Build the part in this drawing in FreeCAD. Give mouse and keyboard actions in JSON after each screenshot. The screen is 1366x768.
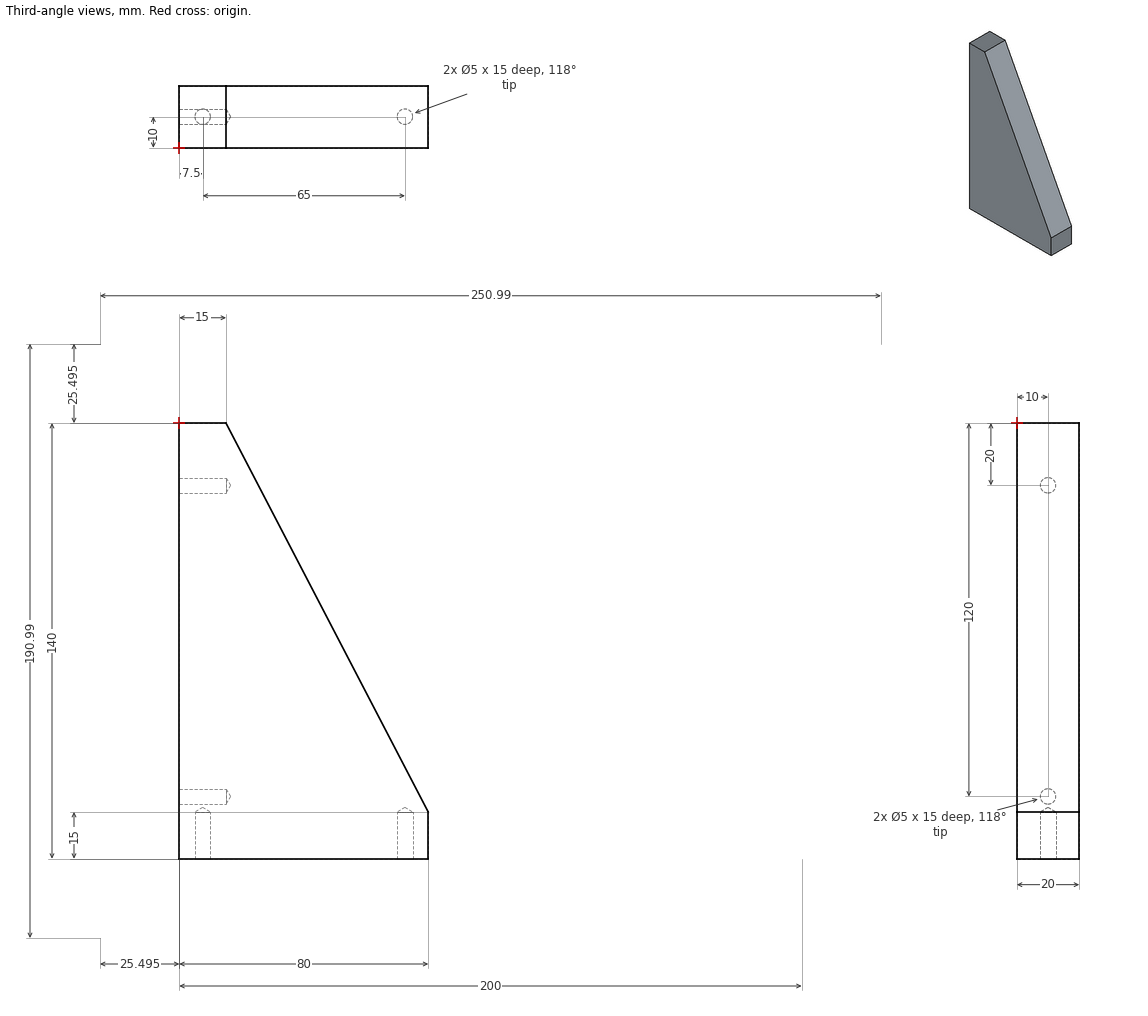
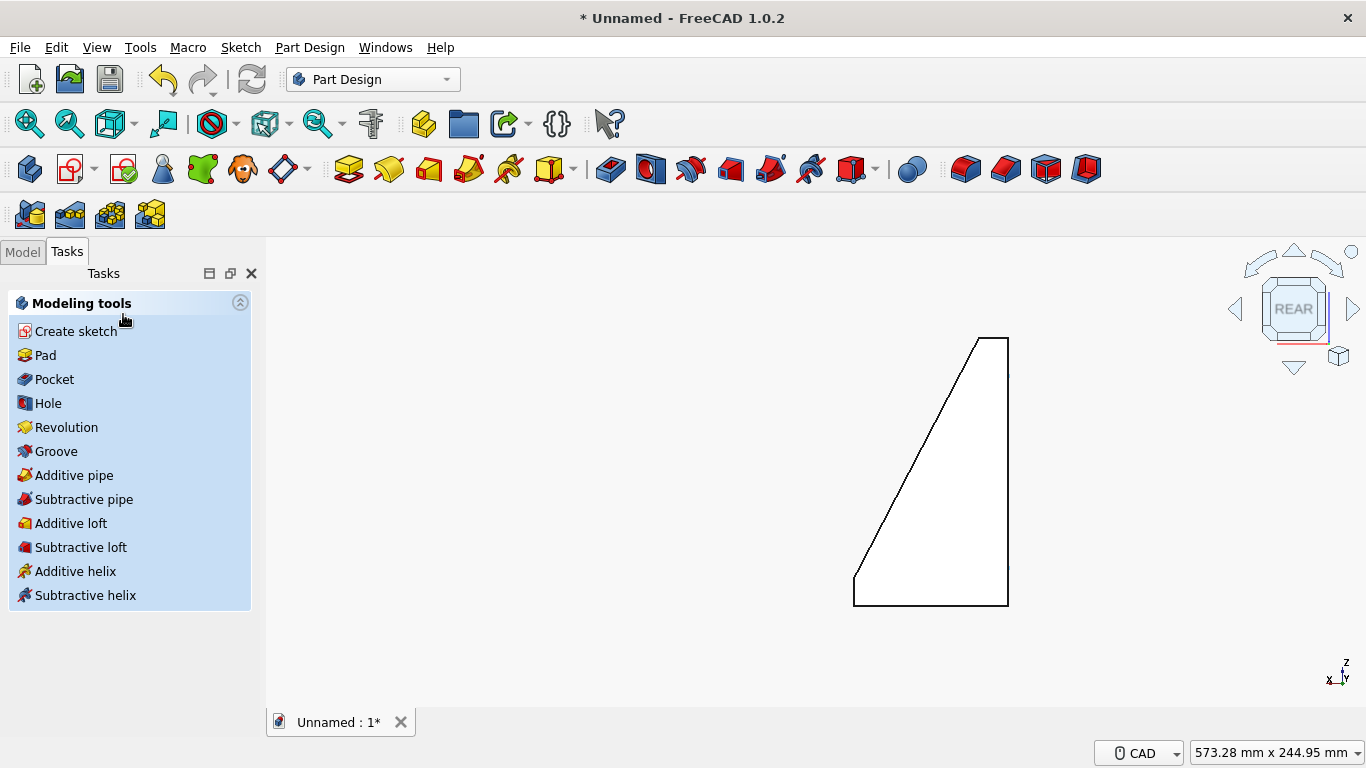
{"action": "left_click", "coordinate": [652, 170]}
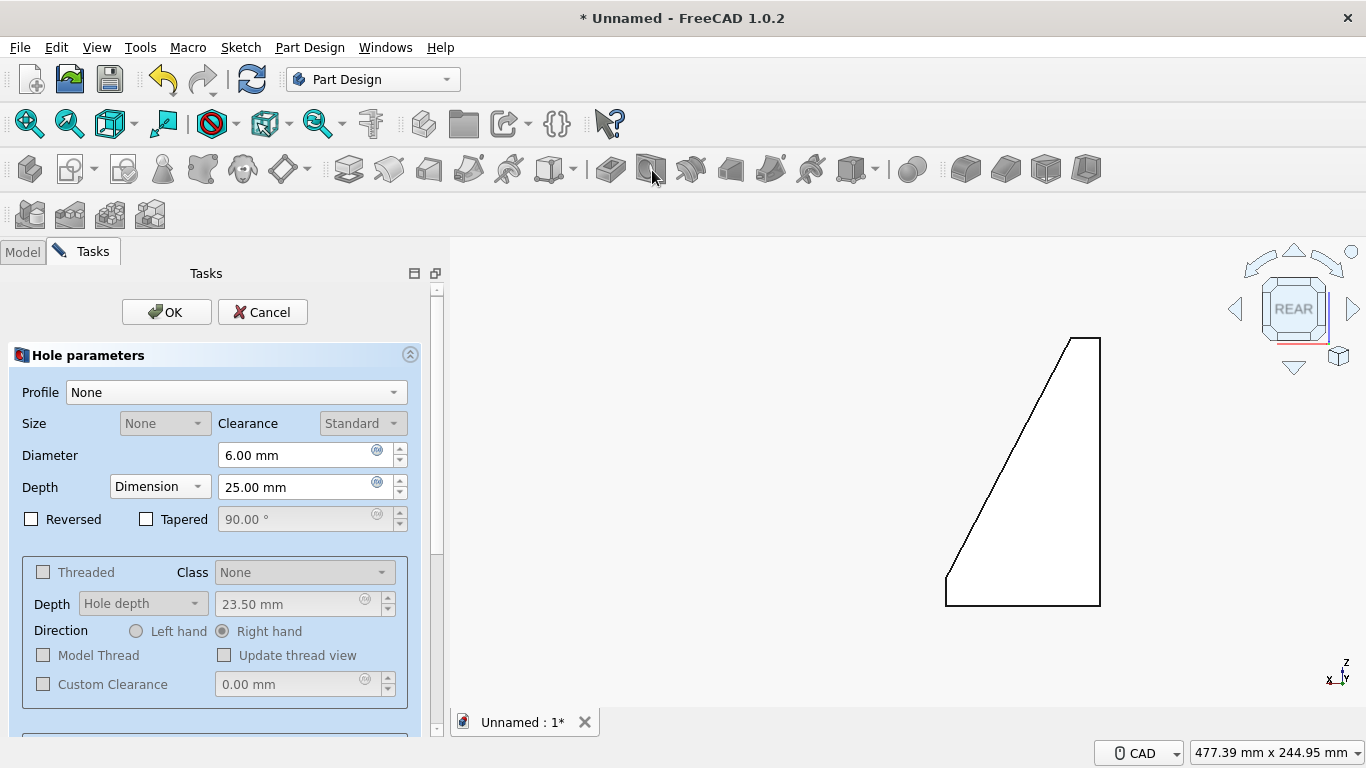
{"action": "triple_click", "coordinate": [305, 455]}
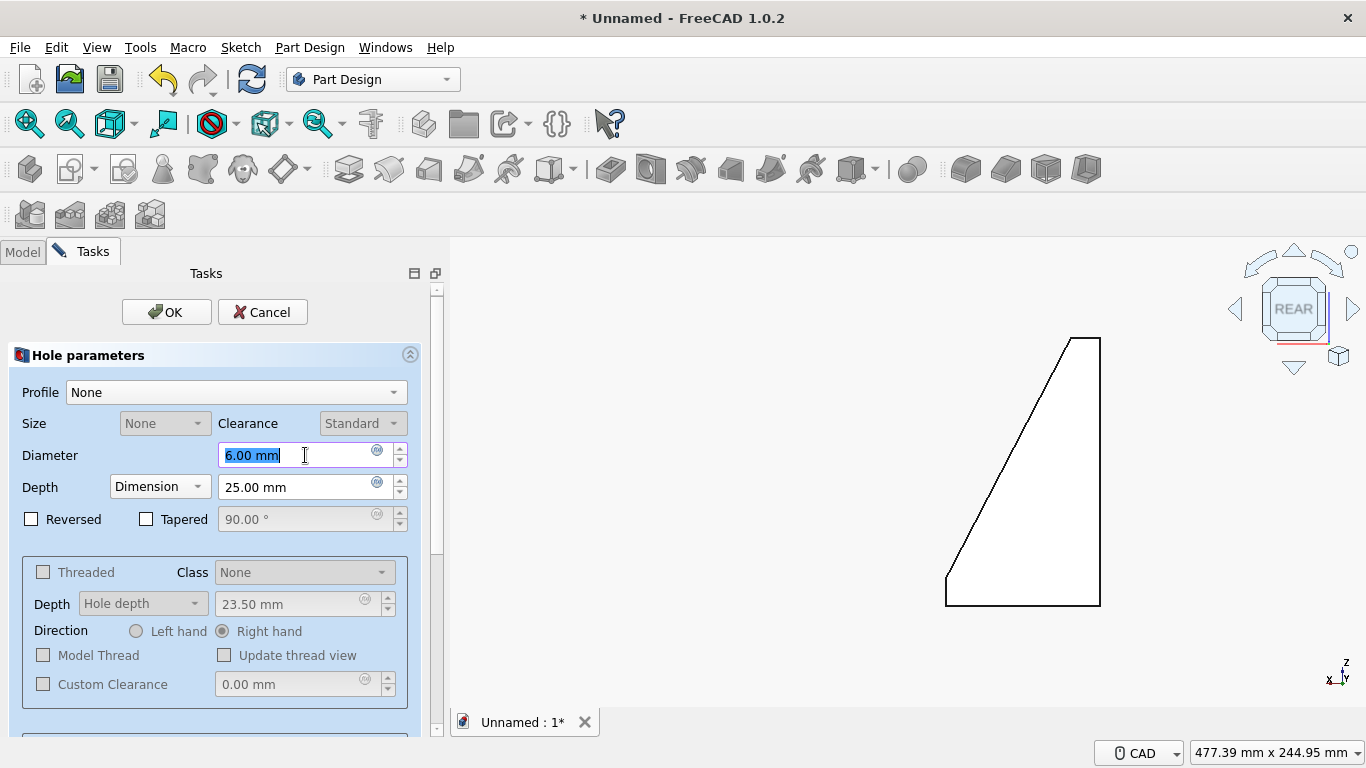
{"action": "type", "text": "5"}
{"action": "key", "text": "Tab"}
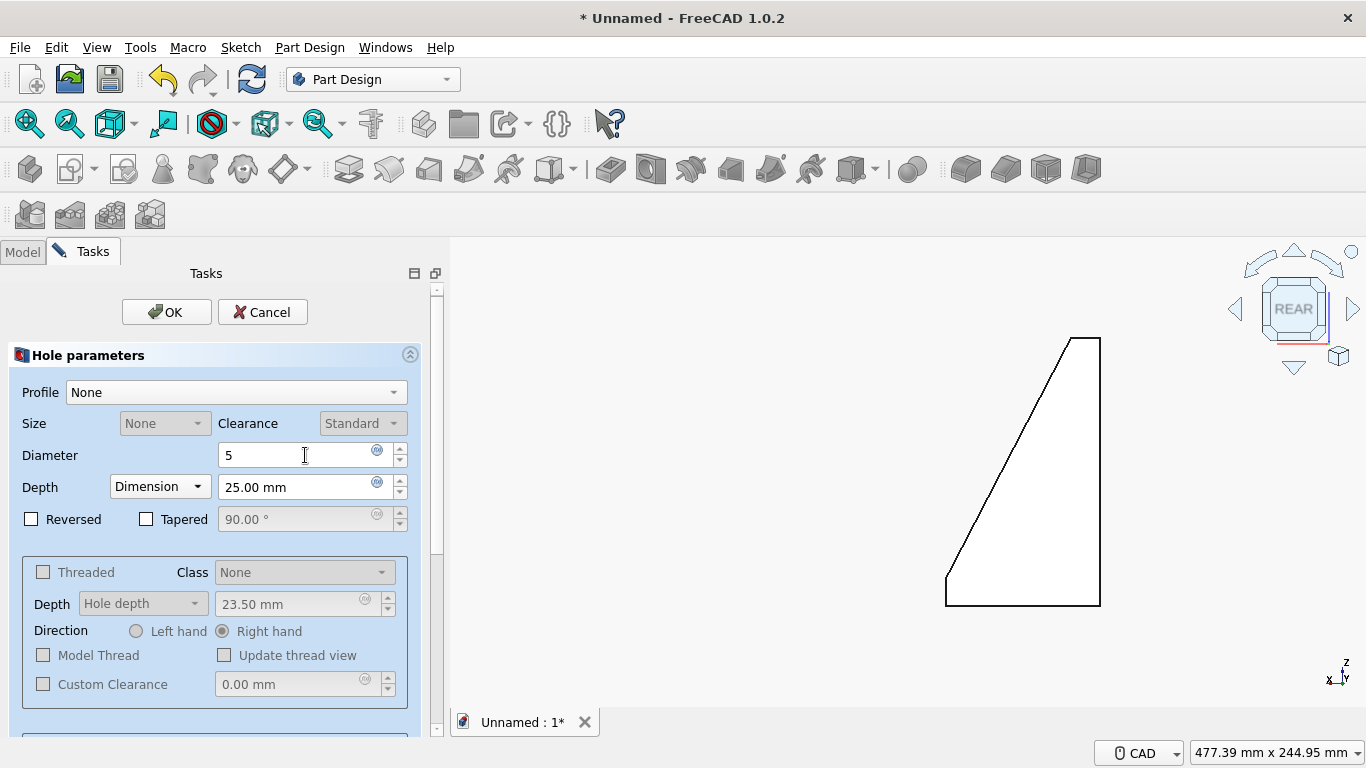
{"action": "triple_click", "coordinate": [305, 487]}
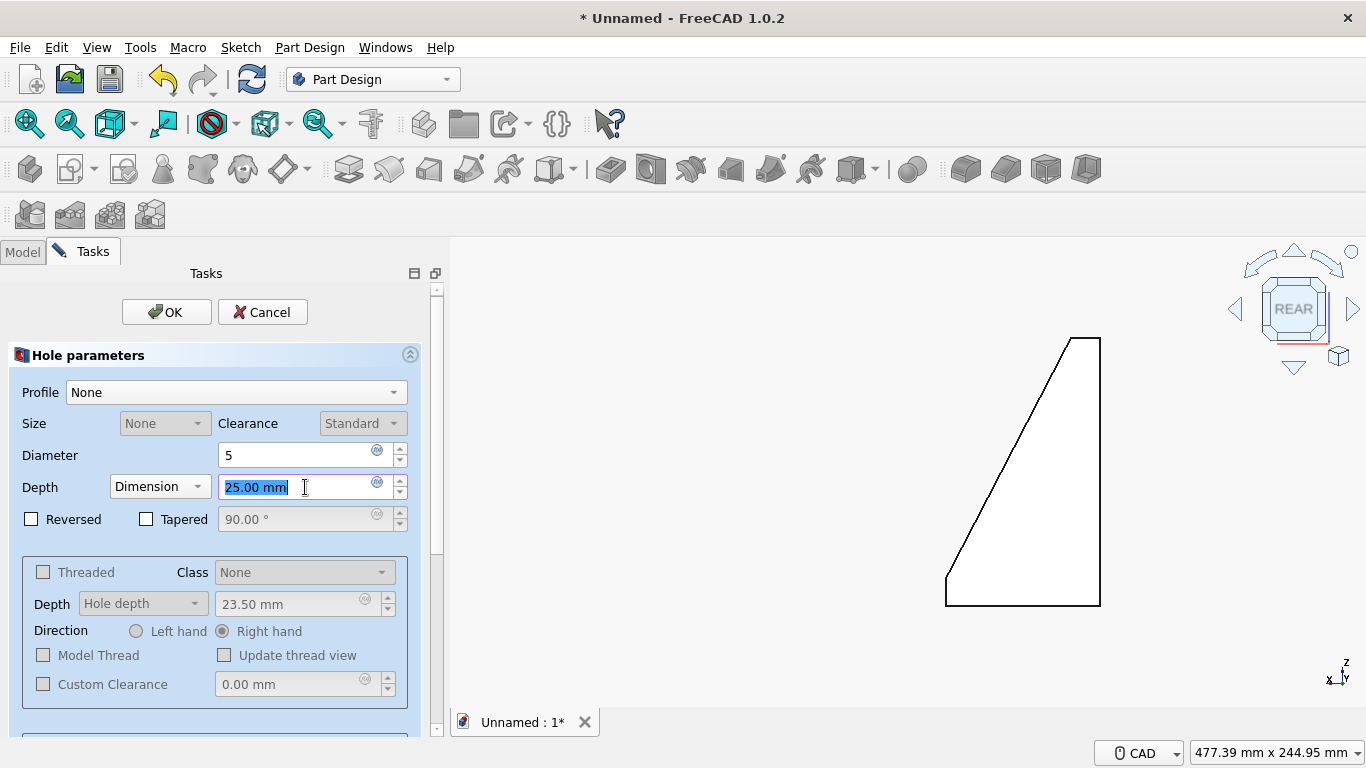
{"action": "type", "text": "15"}
{"action": "key", "text": "Tab"}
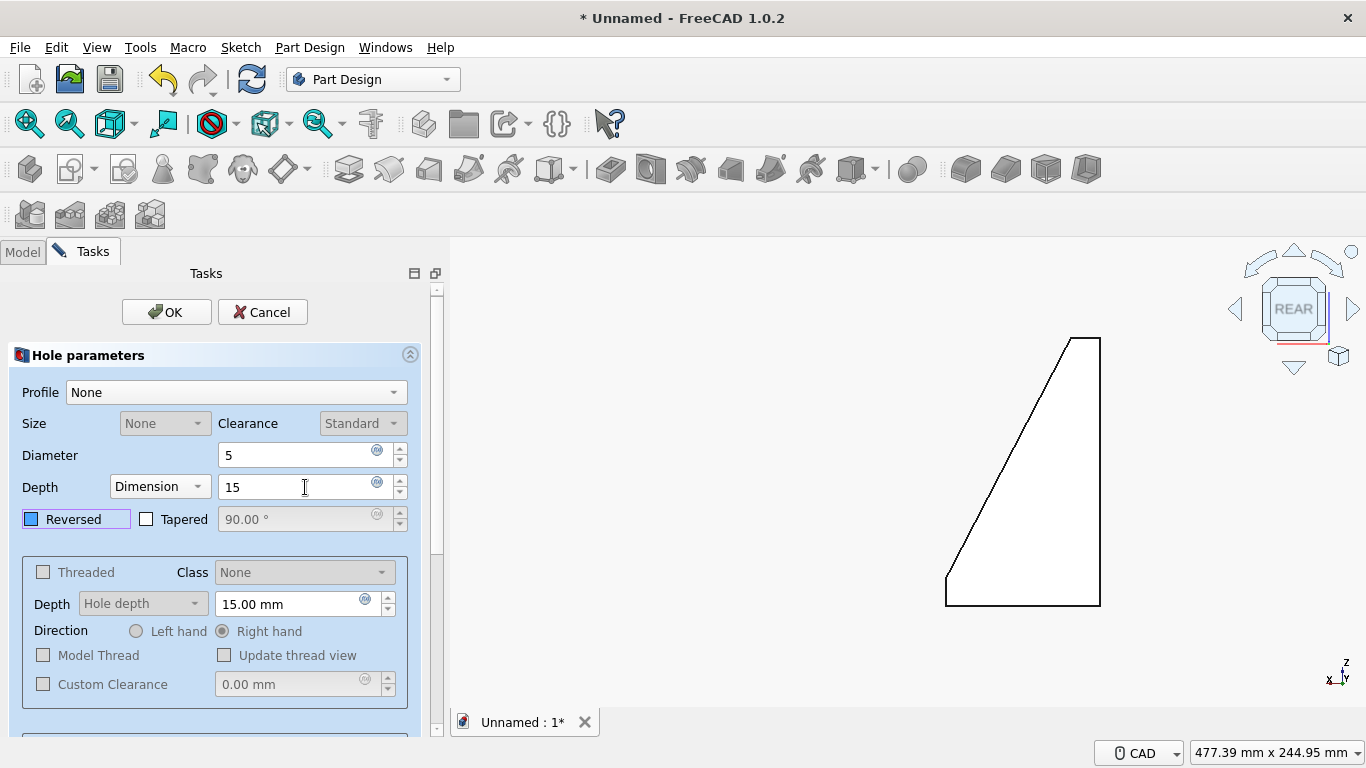
{"action": "left_click", "coordinate": [30, 519]}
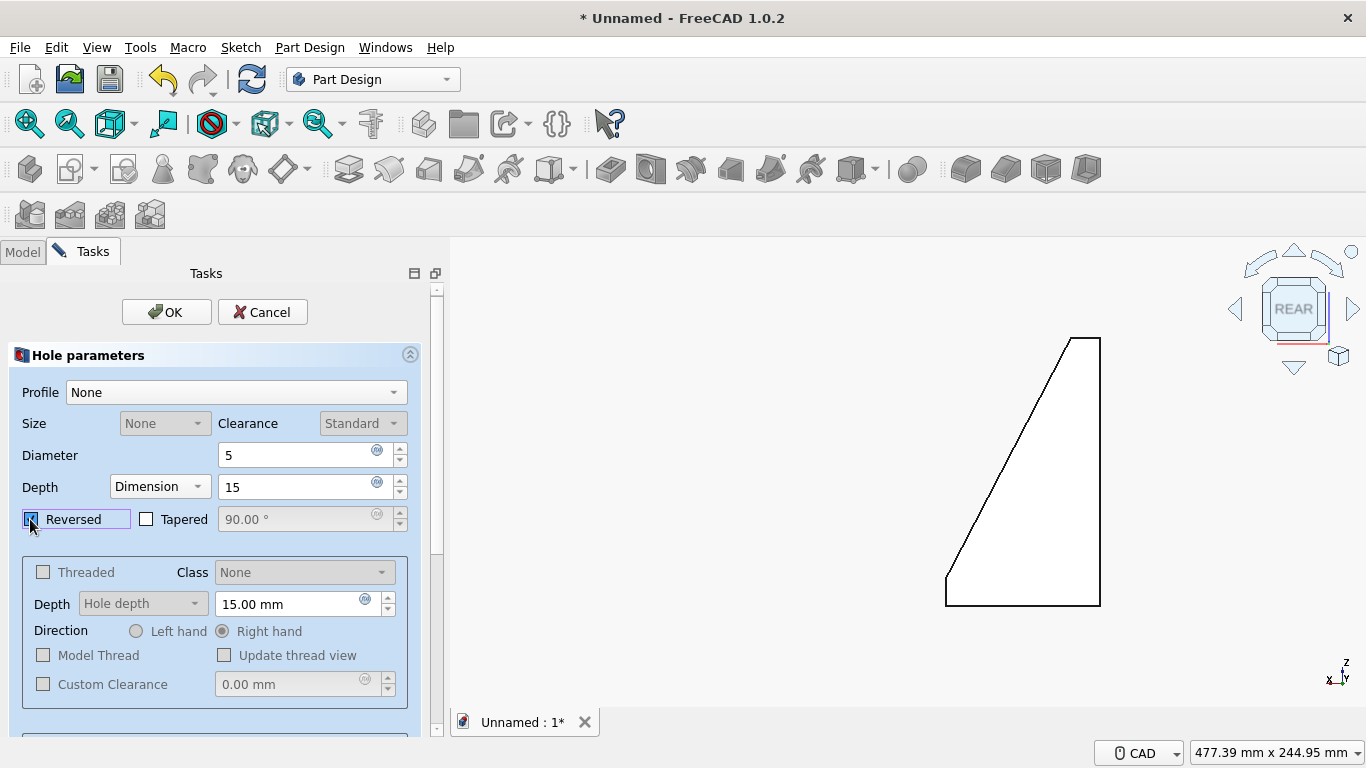
{"action": "left_click", "coordinate": [167, 312]}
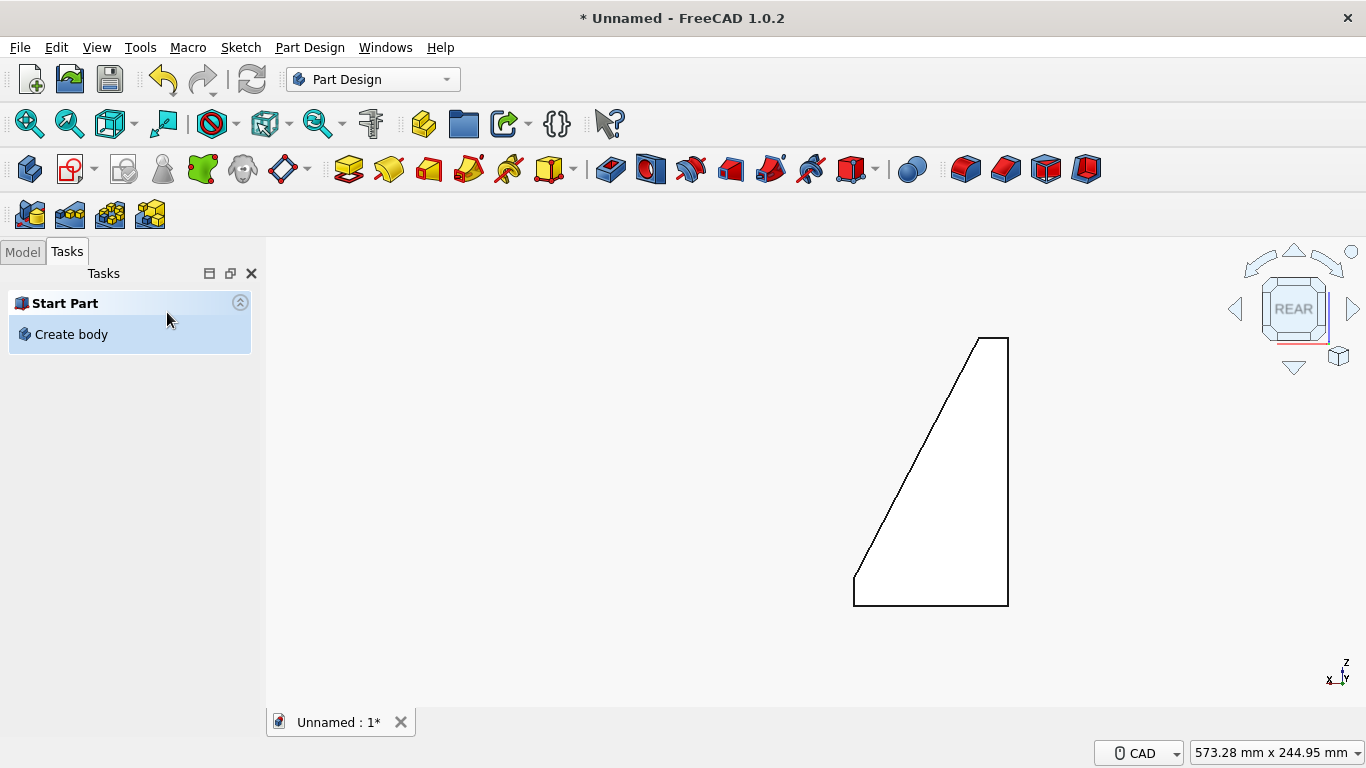
{"action": "key", "text": "5"}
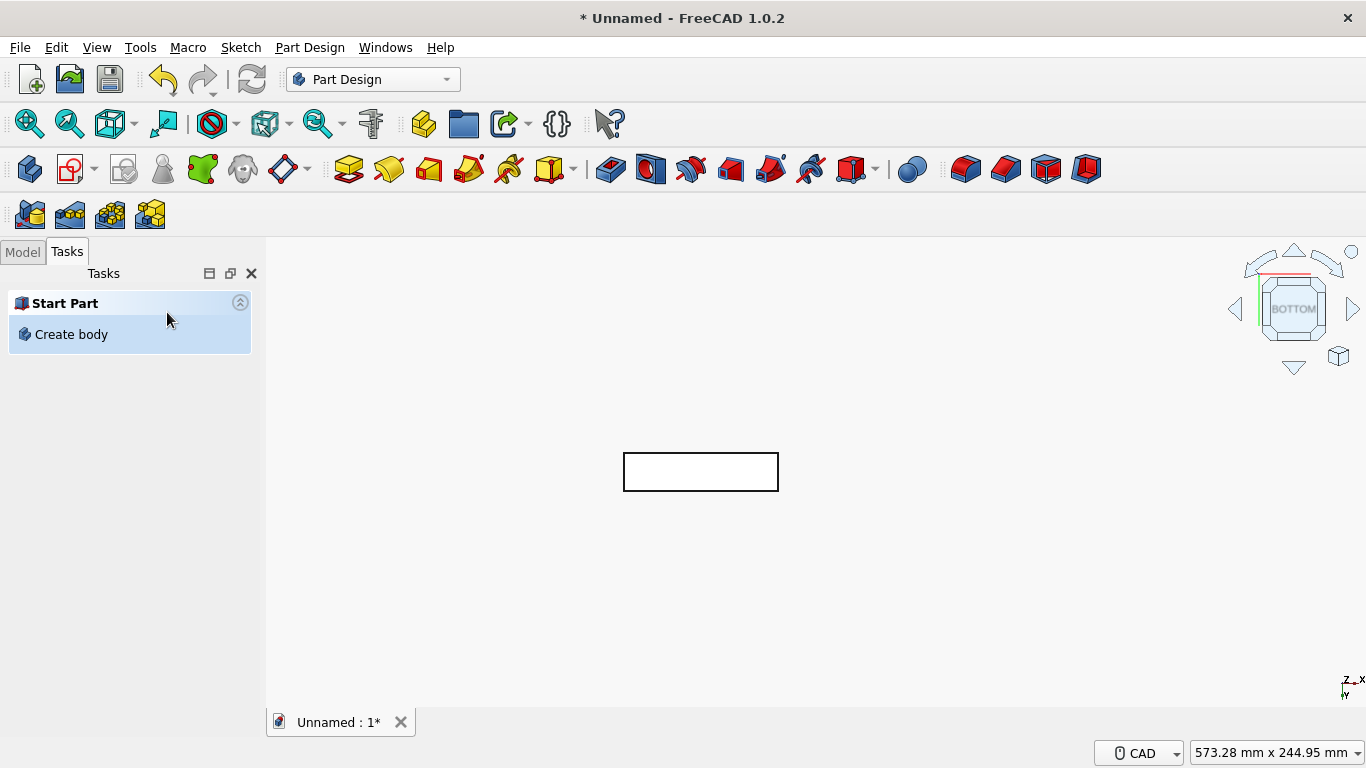
{"action": "left_click", "coordinate": [30, 124]}